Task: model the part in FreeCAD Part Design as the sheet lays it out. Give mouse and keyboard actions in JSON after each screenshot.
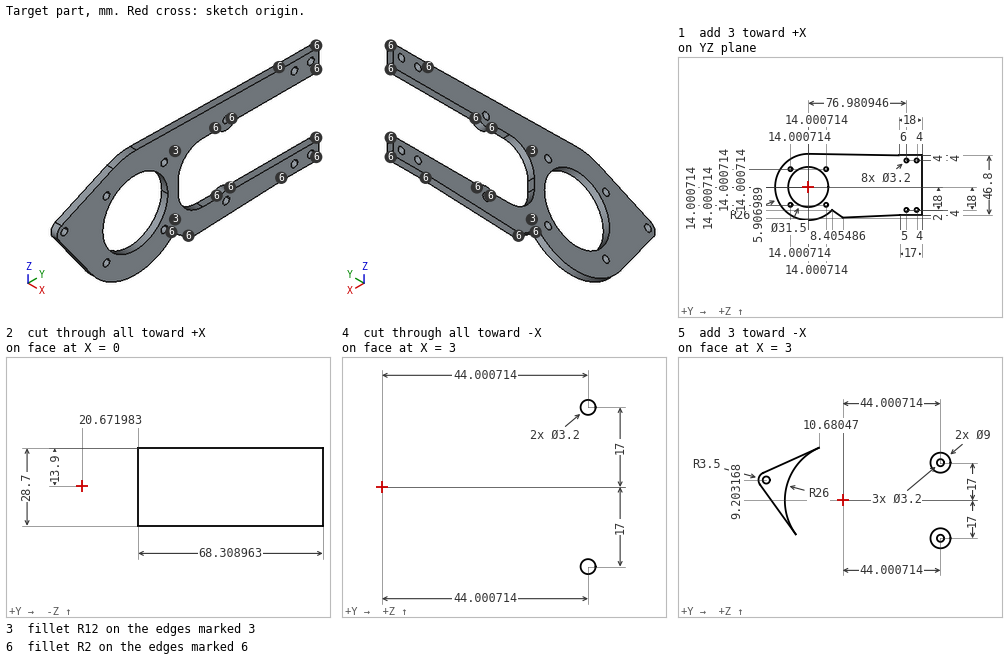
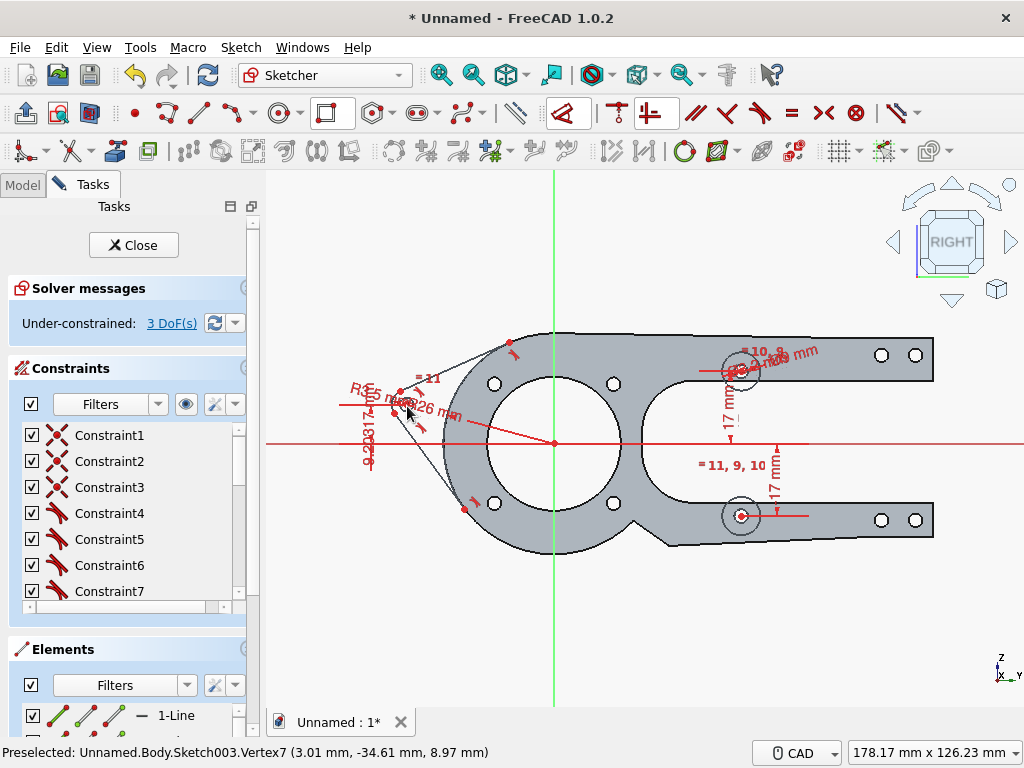
{"action": "left_click", "coordinate": [509, 343]}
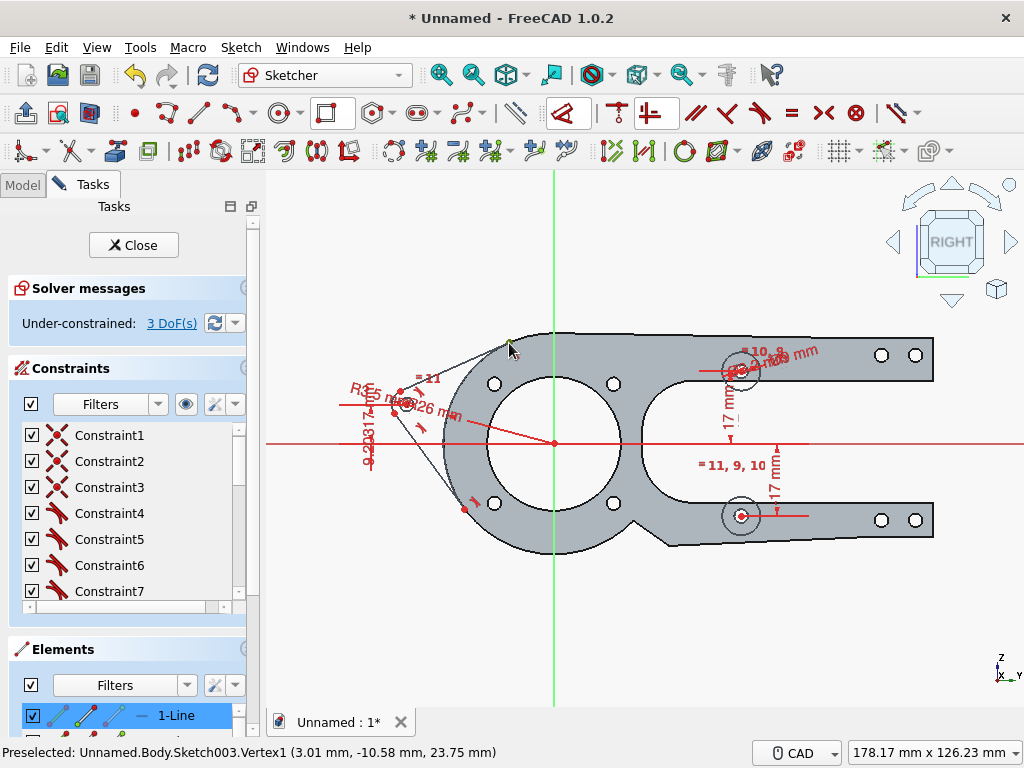
{"action": "left_click", "coordinate": [586, 114]}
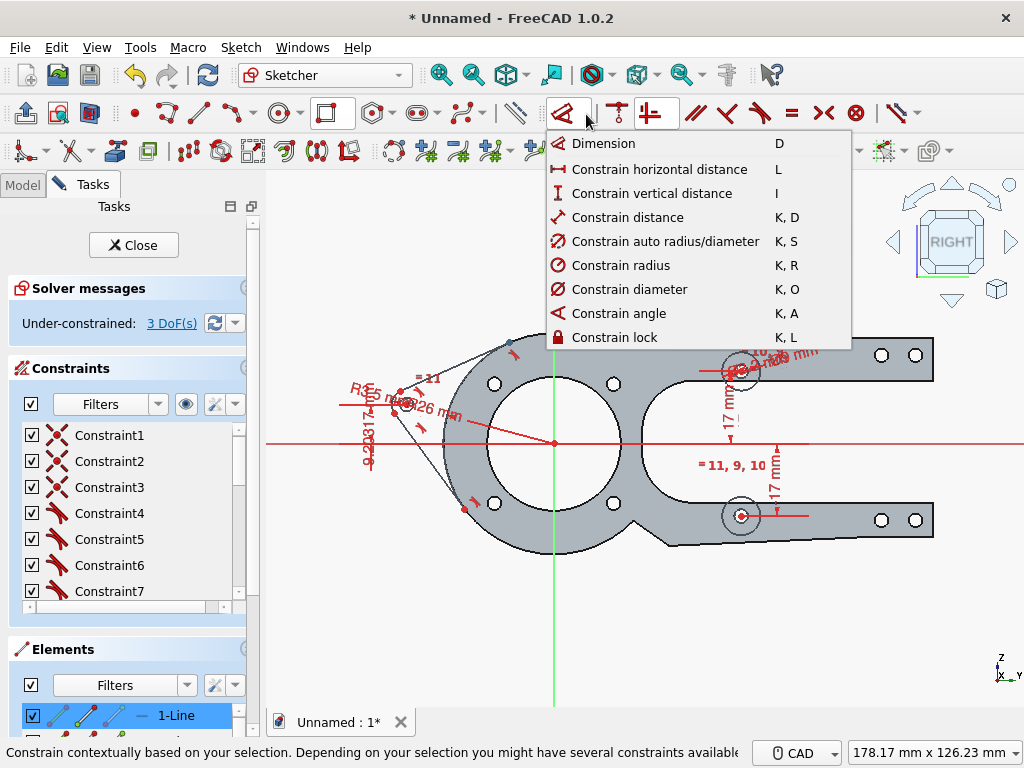
{"action": "left_click", "coordinate": [699, 169]}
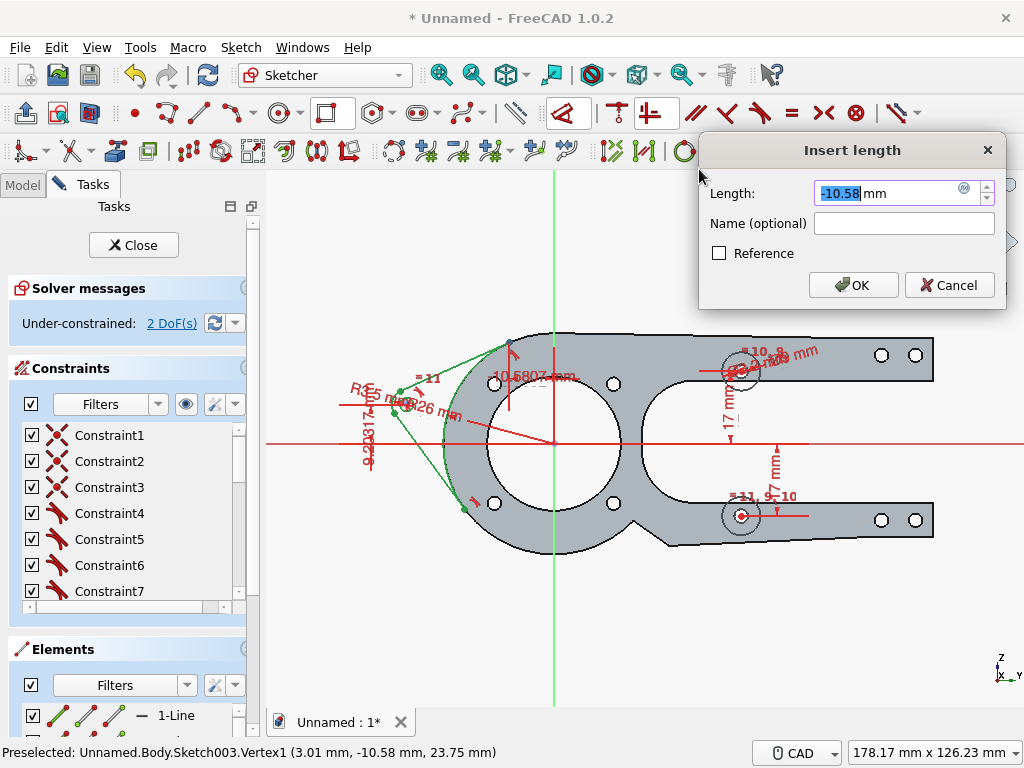
{"action": "type", "text": "-10.68047"}
{"action": "key", "text": "Return"}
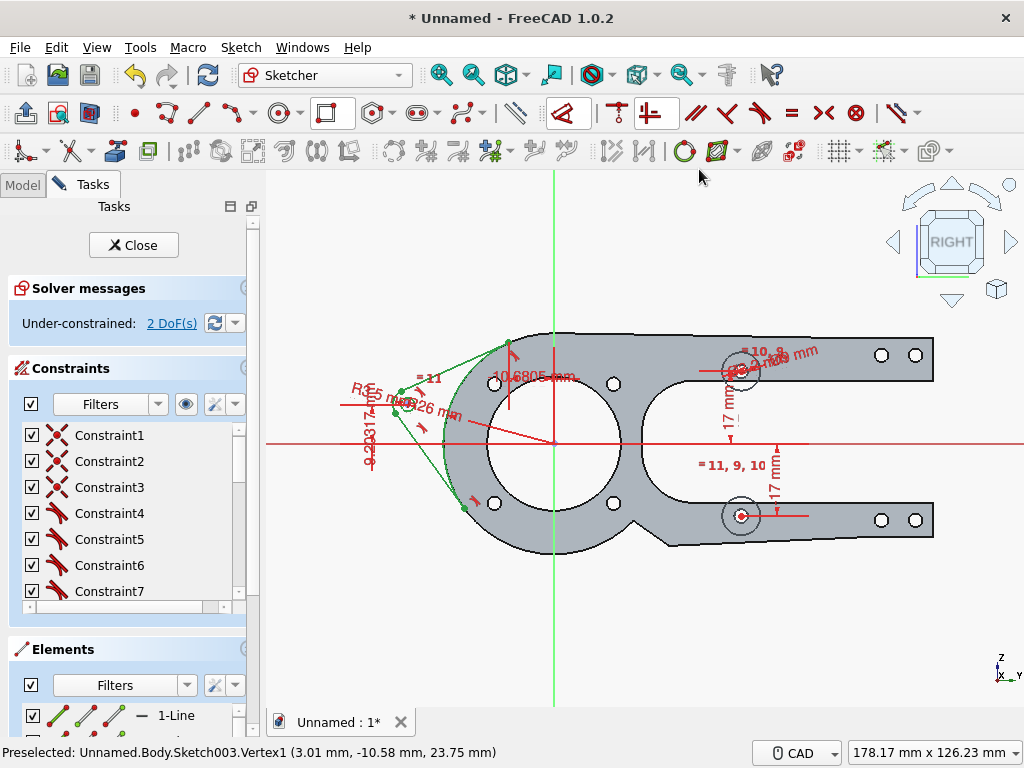
{"action": "left_click", "coordinate": [741, 371]}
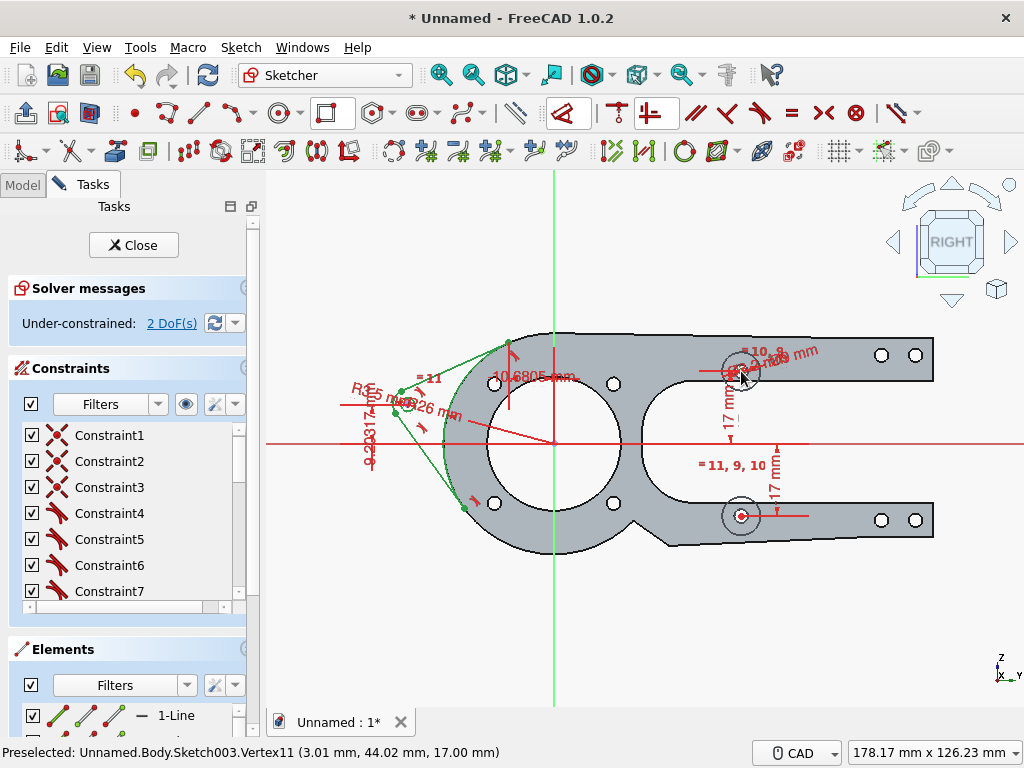
{"action": "left_click", "coordinate": [586, 114]}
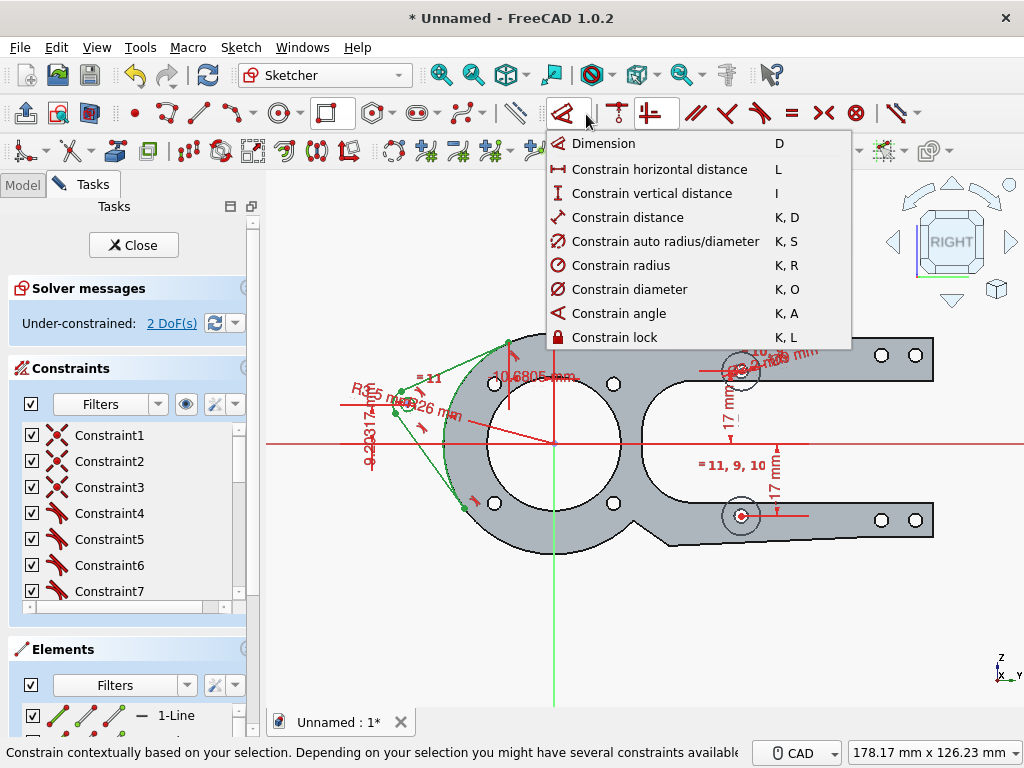
{"action": "left_click", "coordinate": [699, 169]}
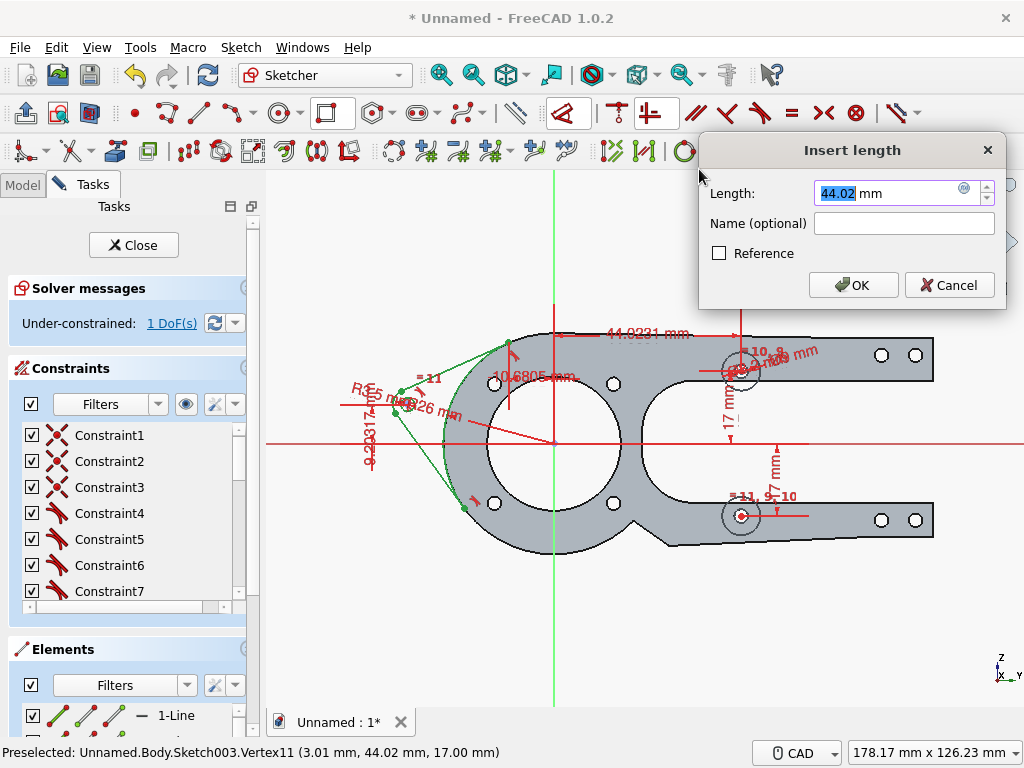
{"action": "type", "text": "44.000714"}
{"action": "key", "text": "Return"}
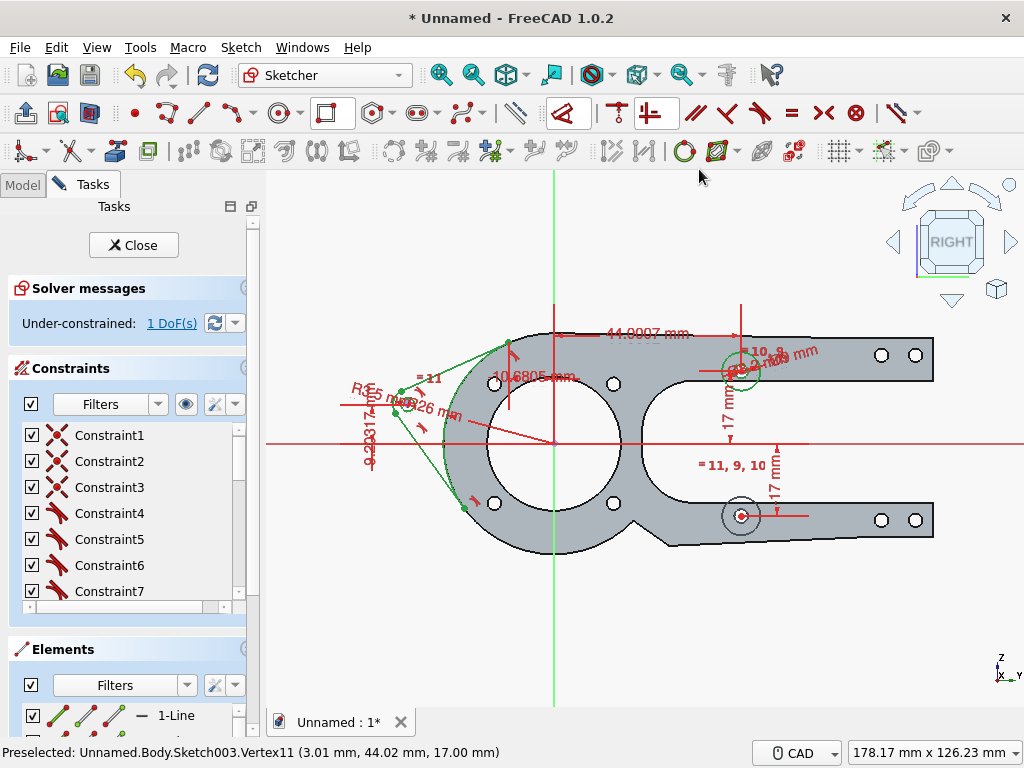
{"action": "left_click", "coordinate": [741, 516]}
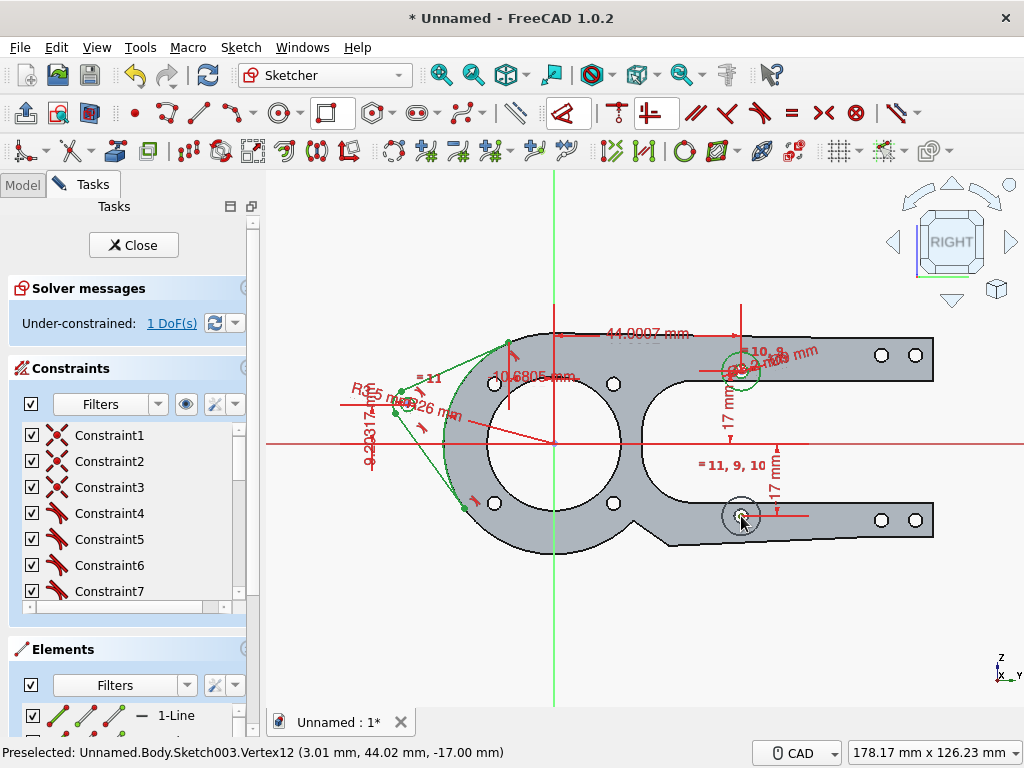
{"action": "left_click", "coordinate": [586, 114]}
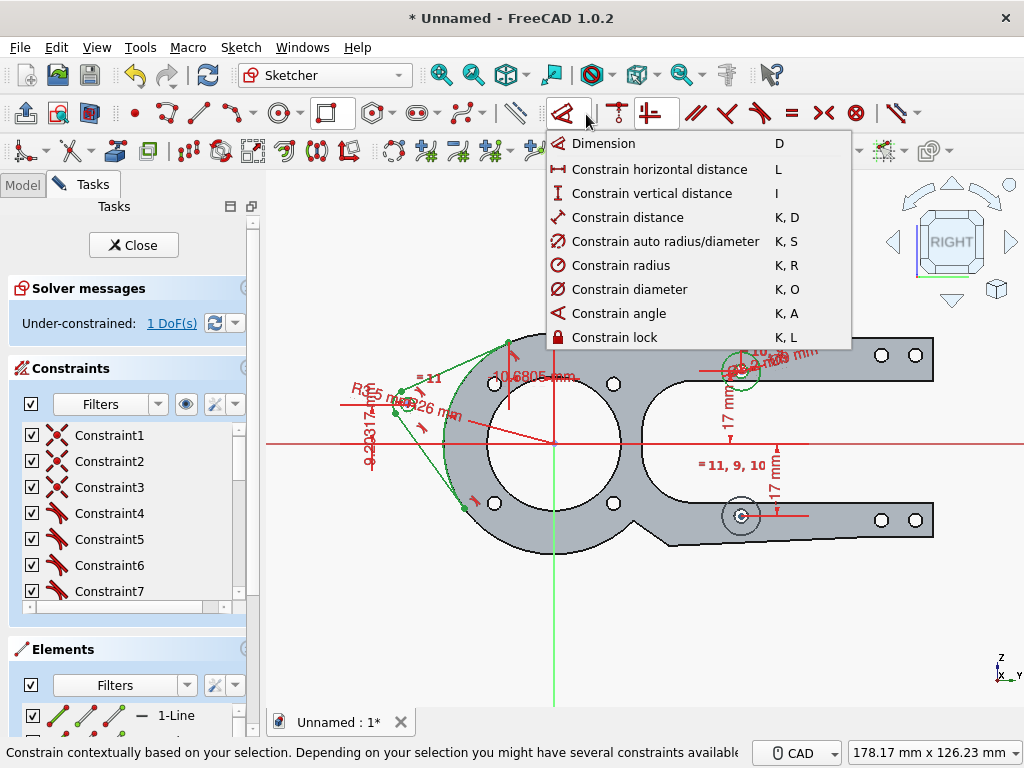
{"action": "left_click", "coordinate": [699, 169]}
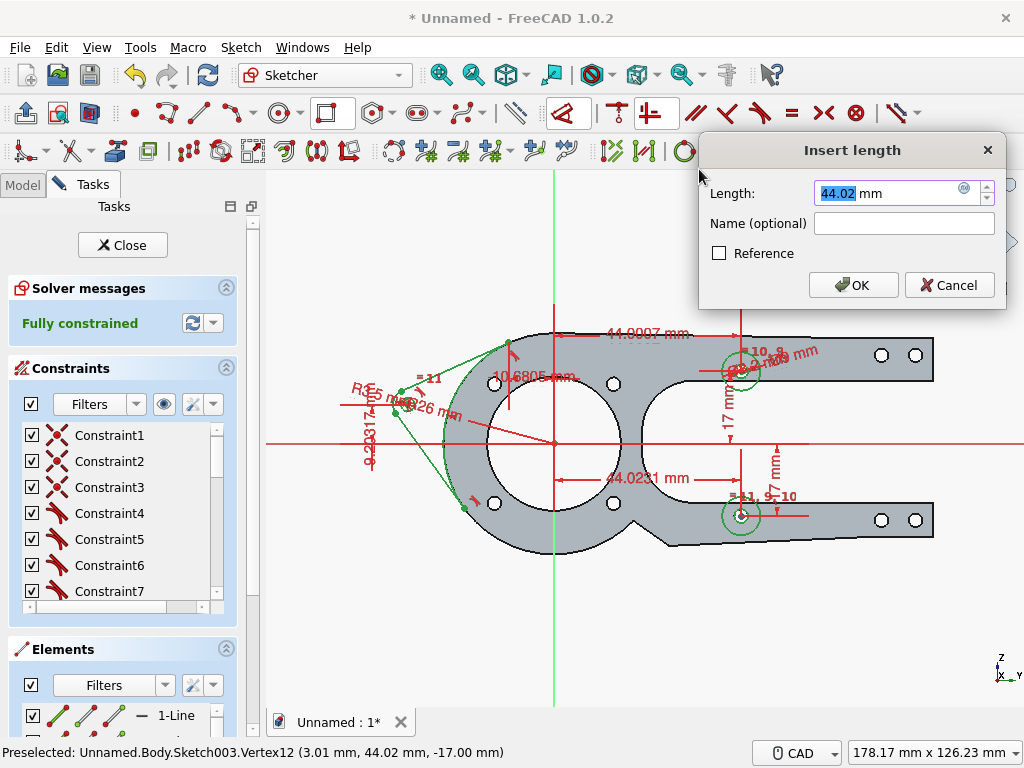
{"action": "type", "text": "44.000714"}
{"action": "key", "text": "Return"}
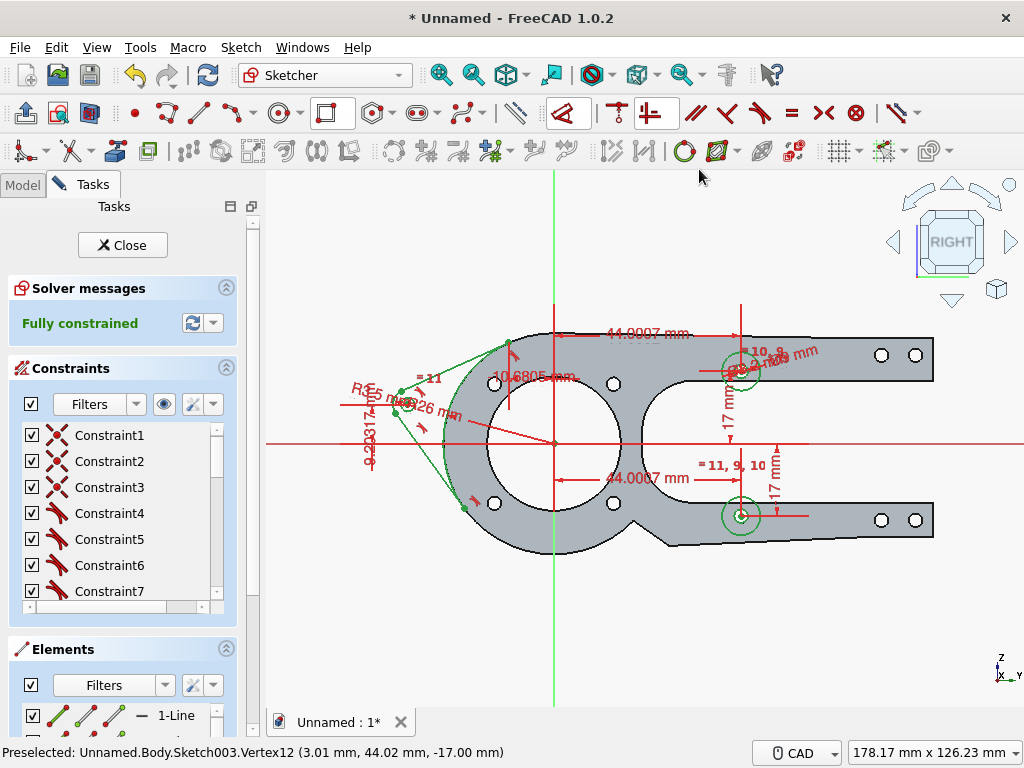
{"action": "left_click", "coordinate": [123, 245]}